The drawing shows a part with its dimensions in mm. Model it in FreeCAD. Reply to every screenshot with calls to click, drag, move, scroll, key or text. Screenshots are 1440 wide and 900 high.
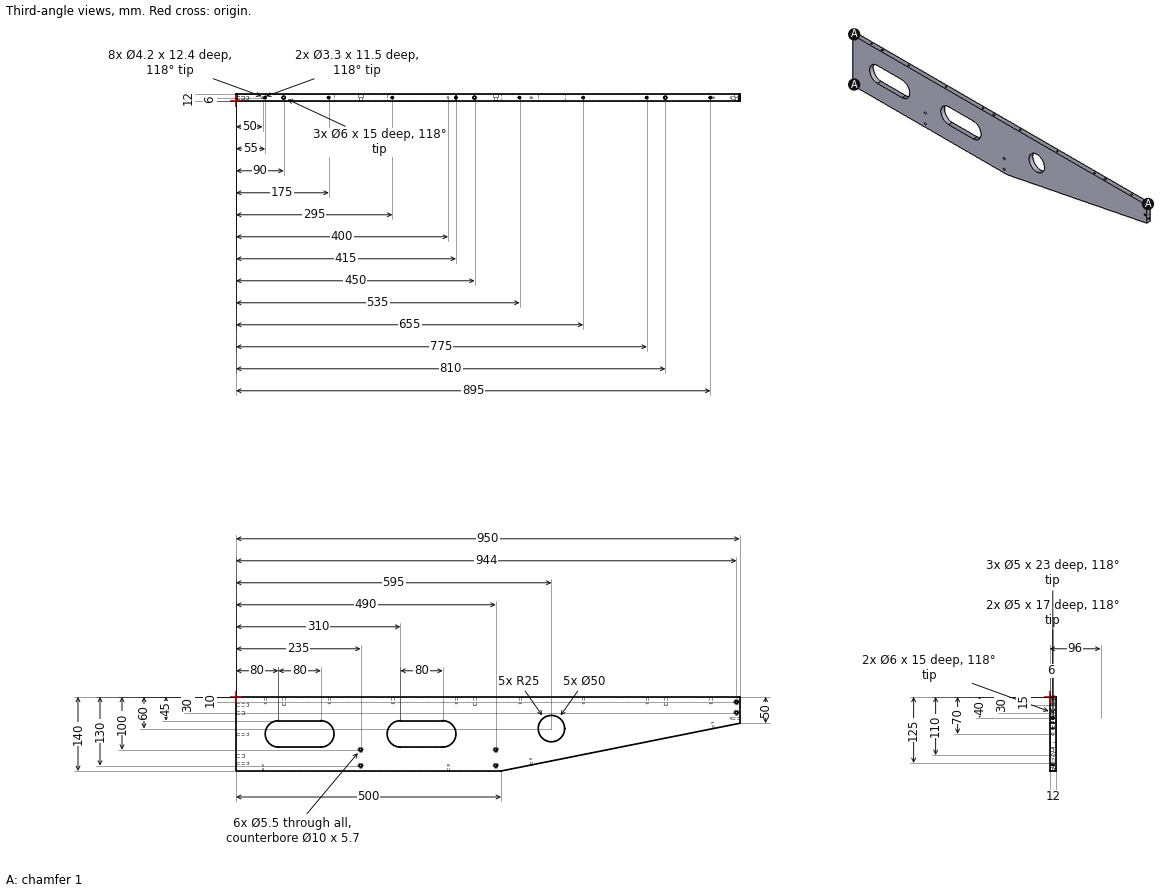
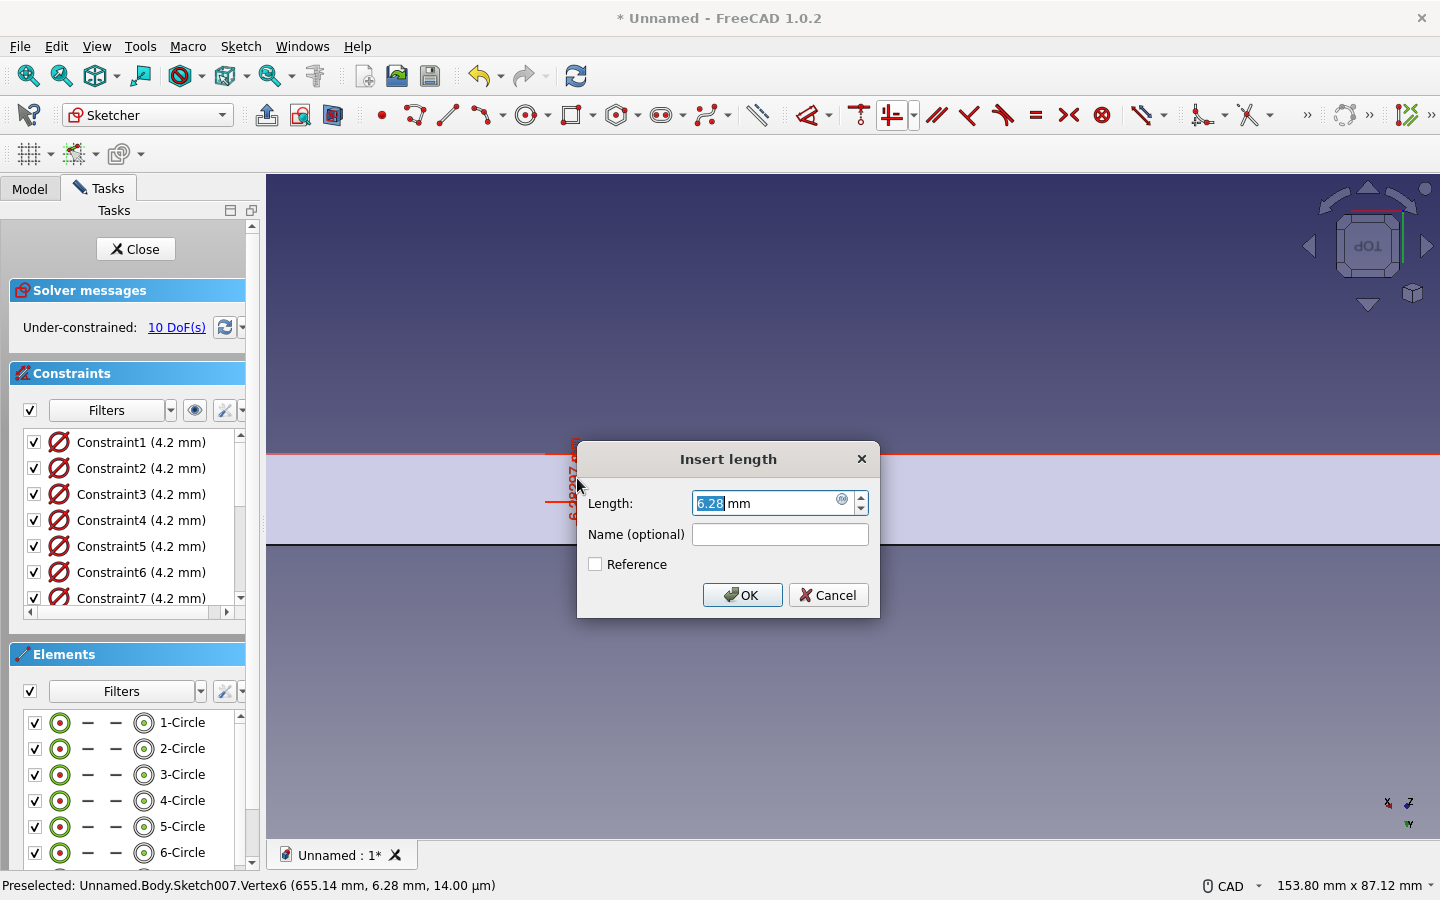
text(6)
key(Return)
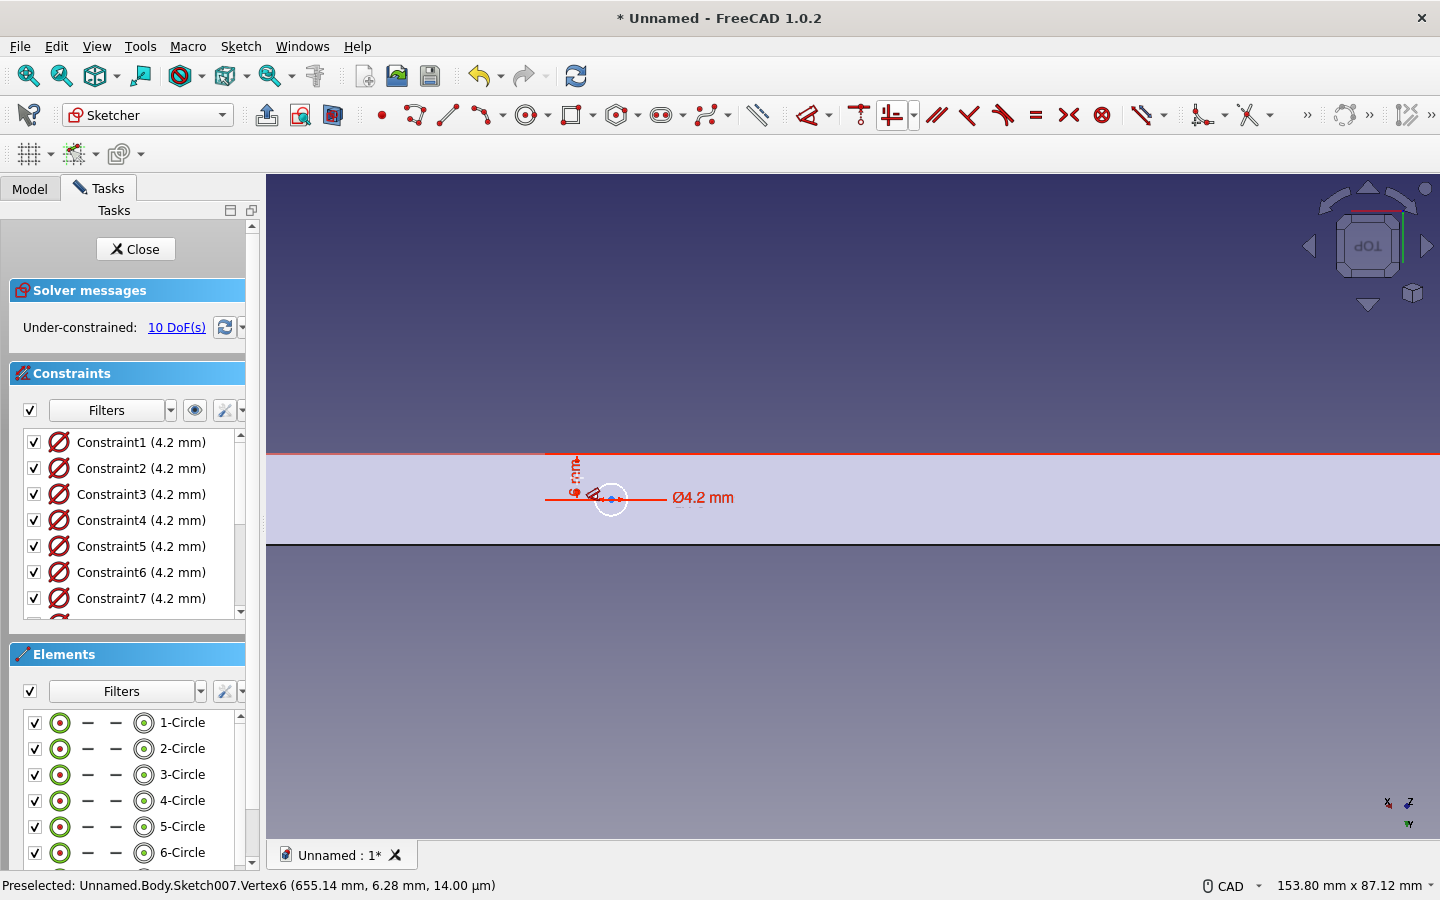
scroll(610, 509, down, 11)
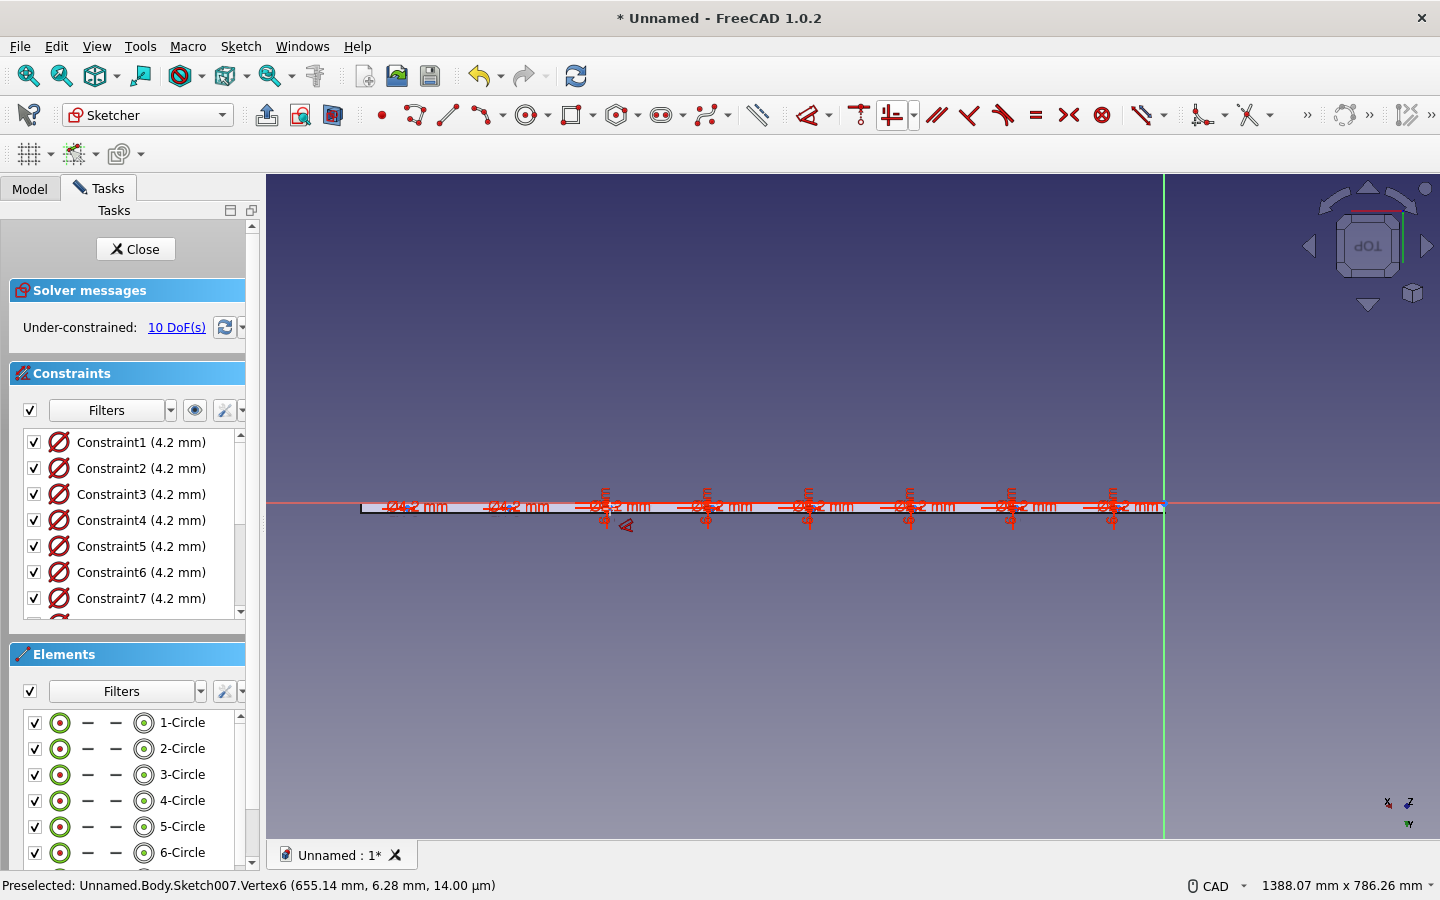
scroll(509, 509, up, 11)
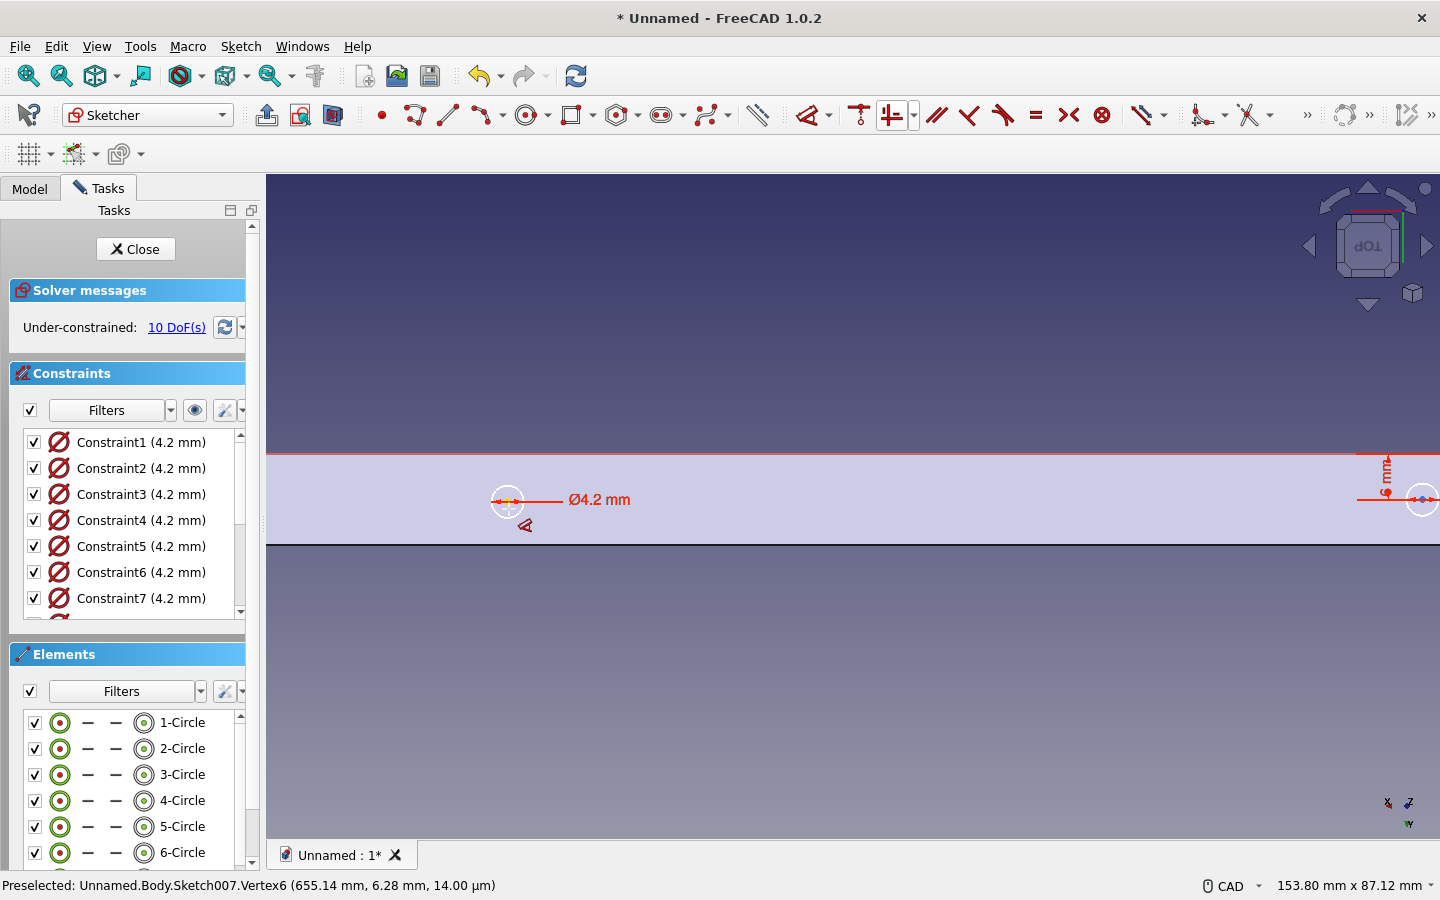
click(508, 502)
click(474, 478)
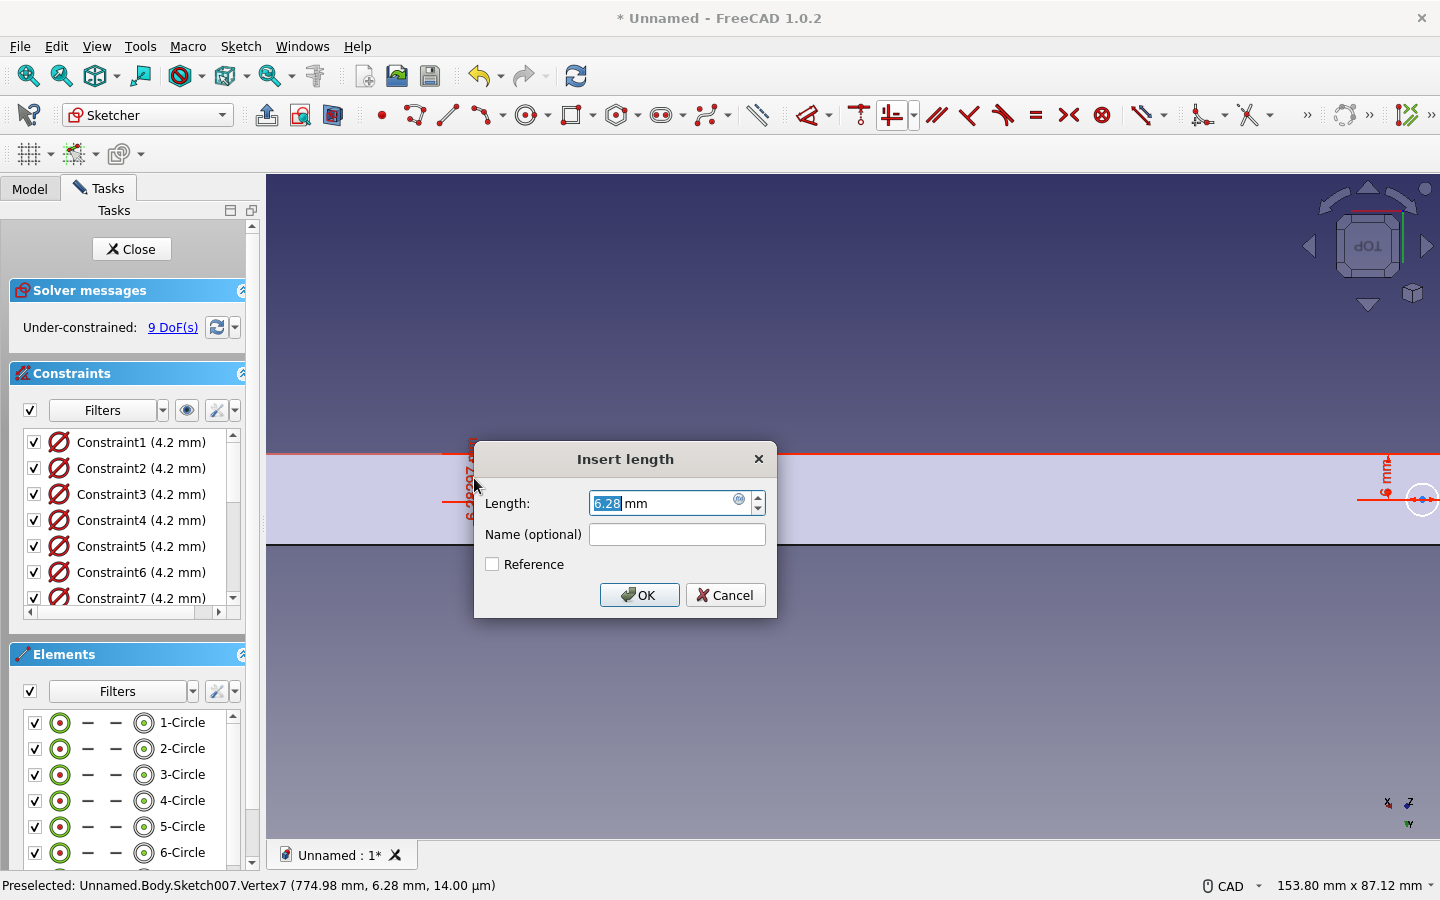
text(6)
key(Return)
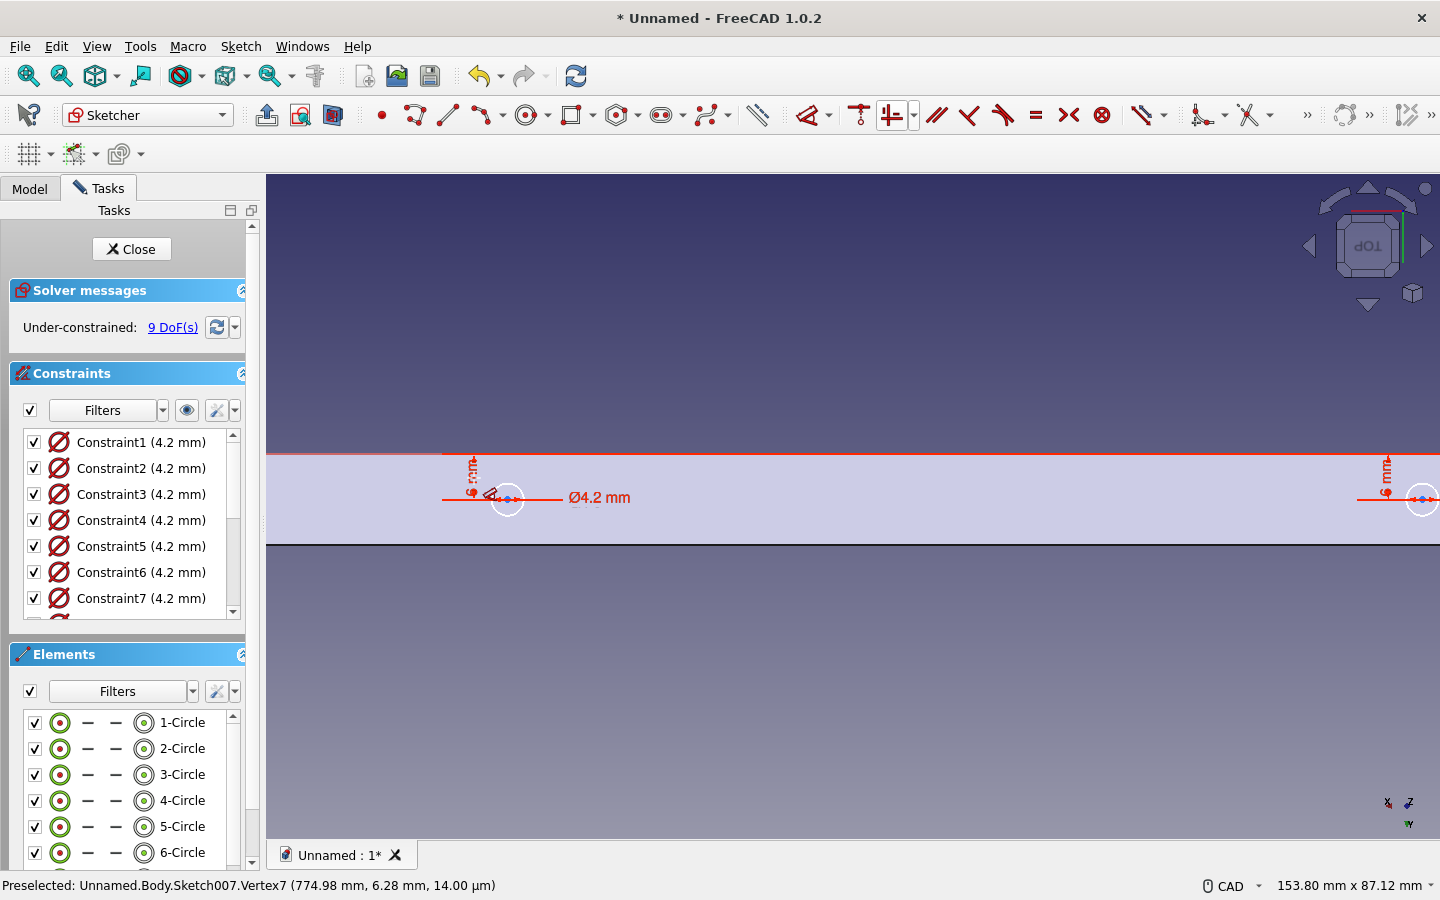
scroll(509, 509, down, 11)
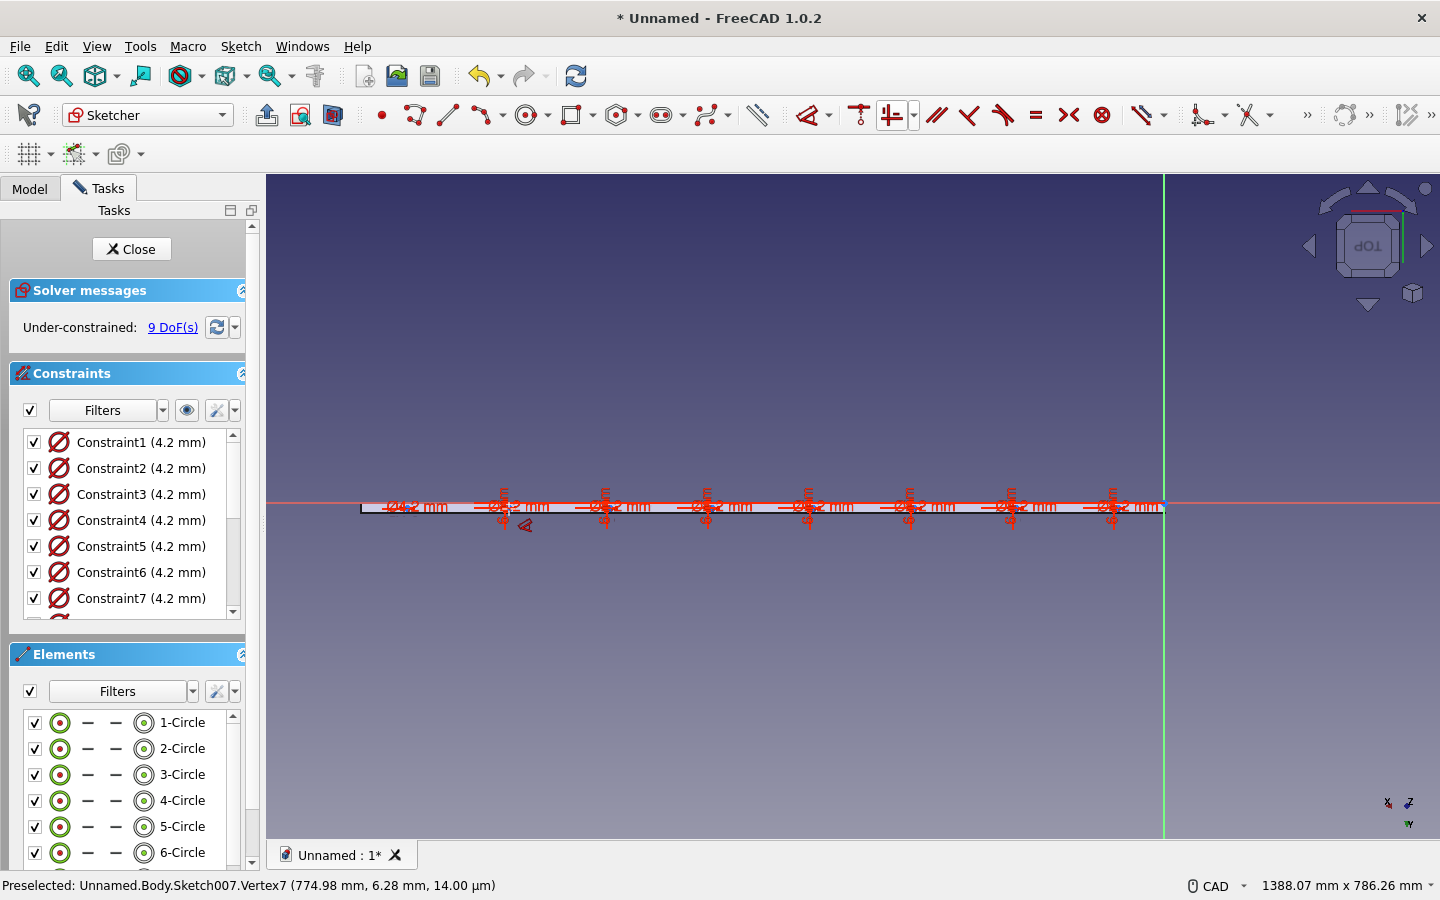
scroll(408, 509, up, 11)